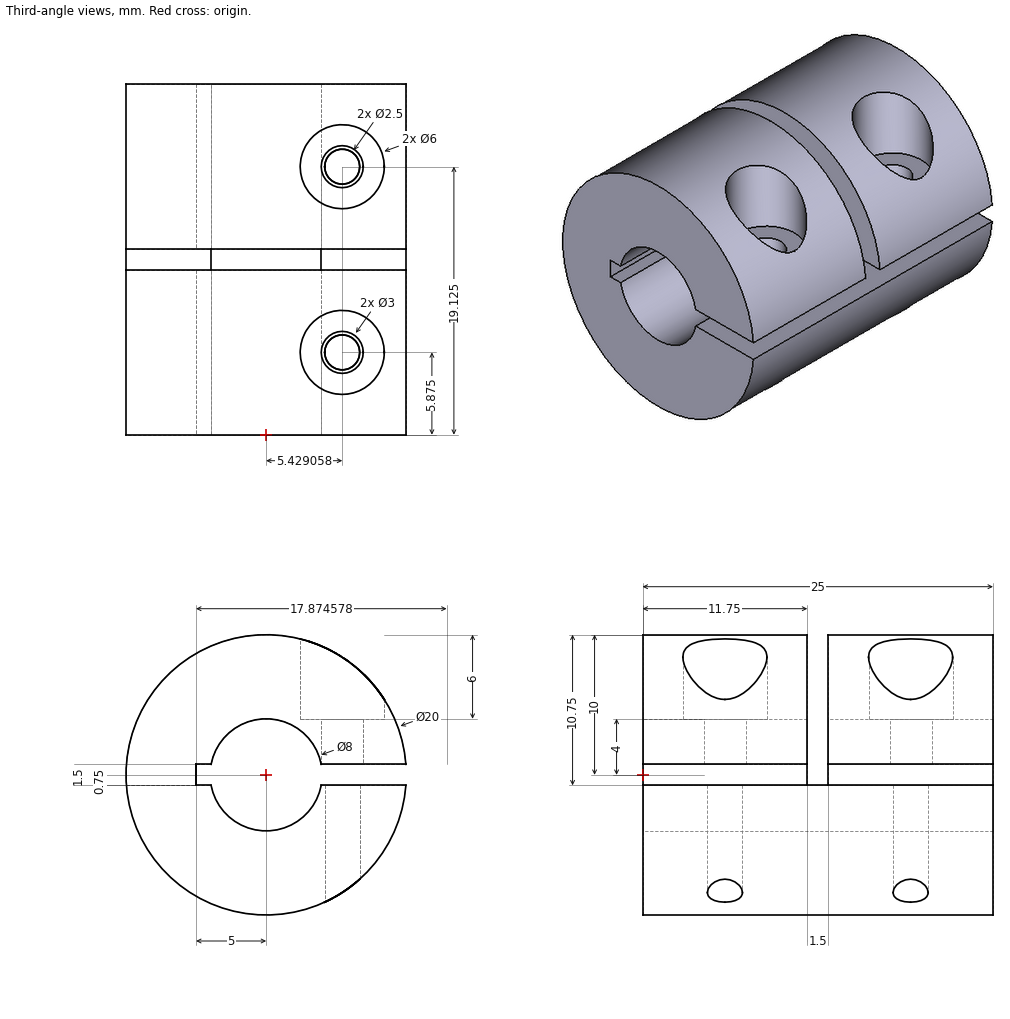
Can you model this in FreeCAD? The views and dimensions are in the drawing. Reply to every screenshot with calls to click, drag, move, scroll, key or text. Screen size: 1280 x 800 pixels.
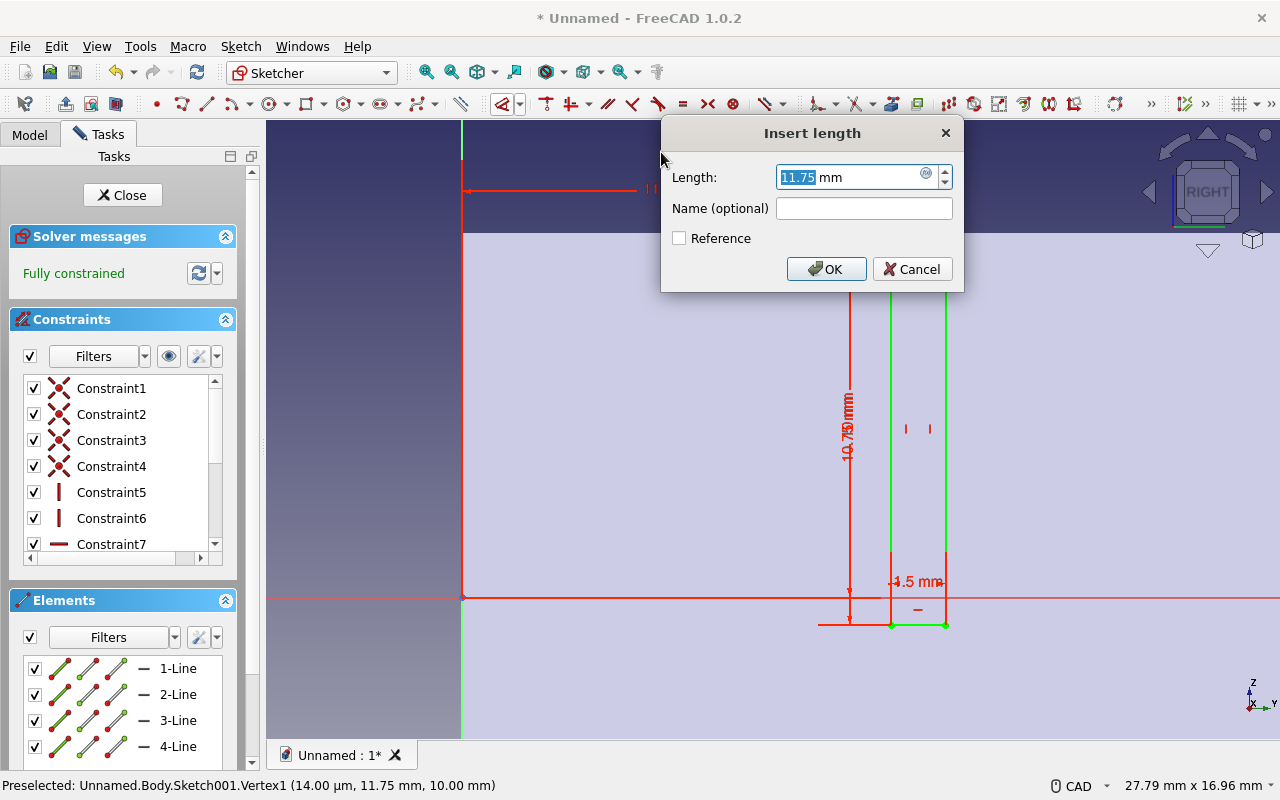
text(11.75)
key(Return)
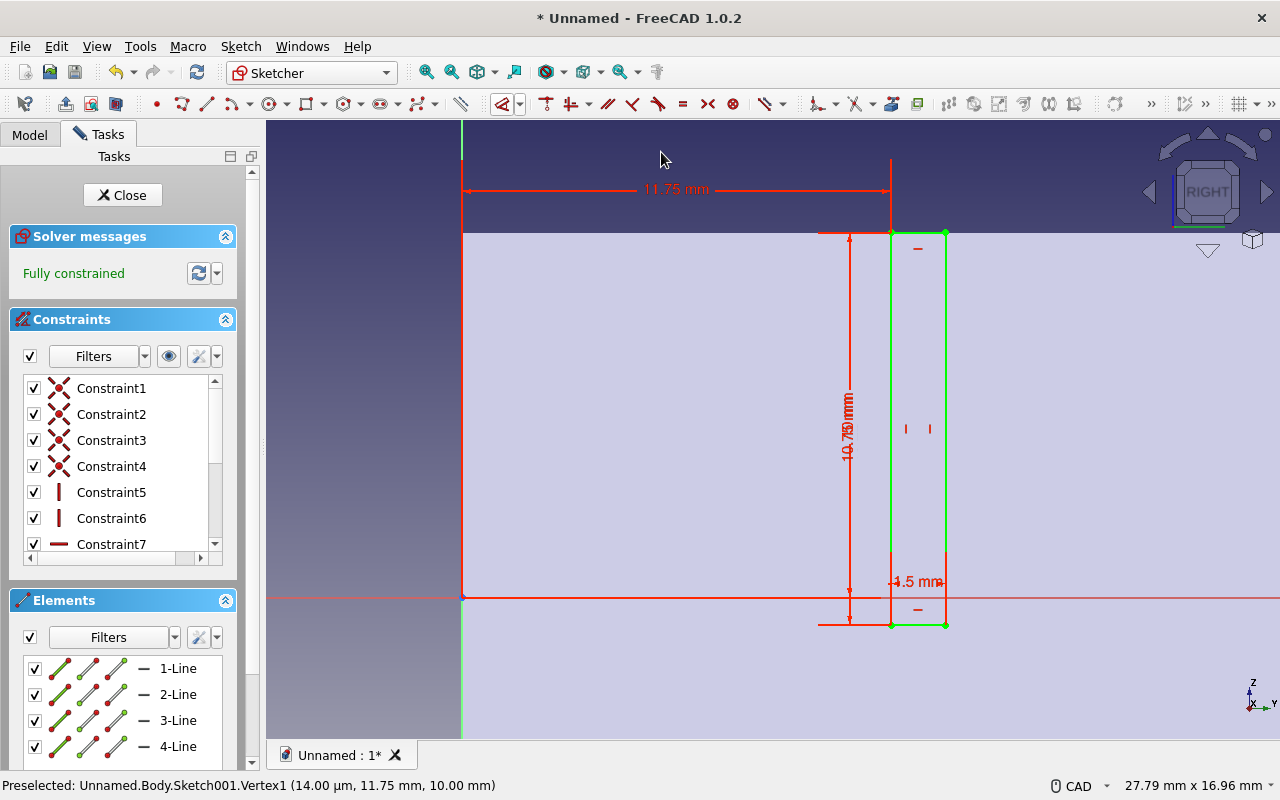
click(123, 195)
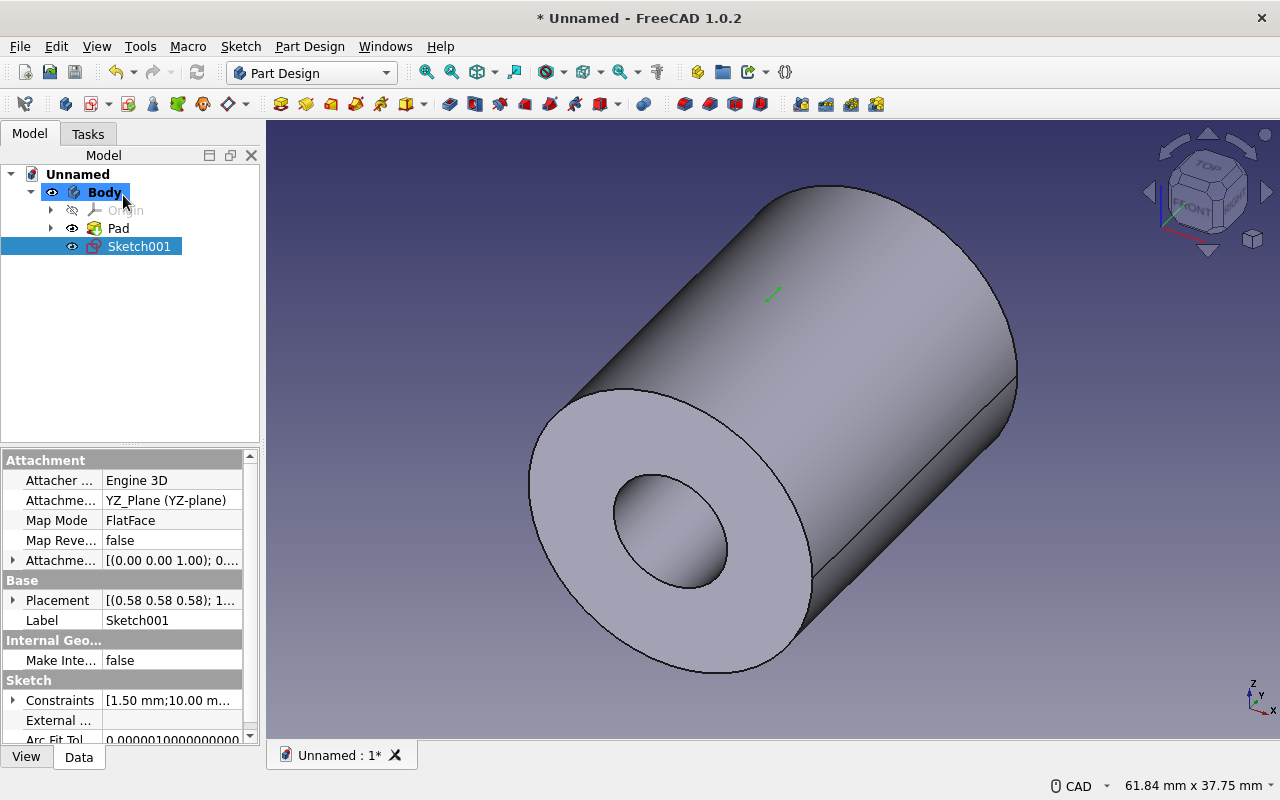
click(450, 104)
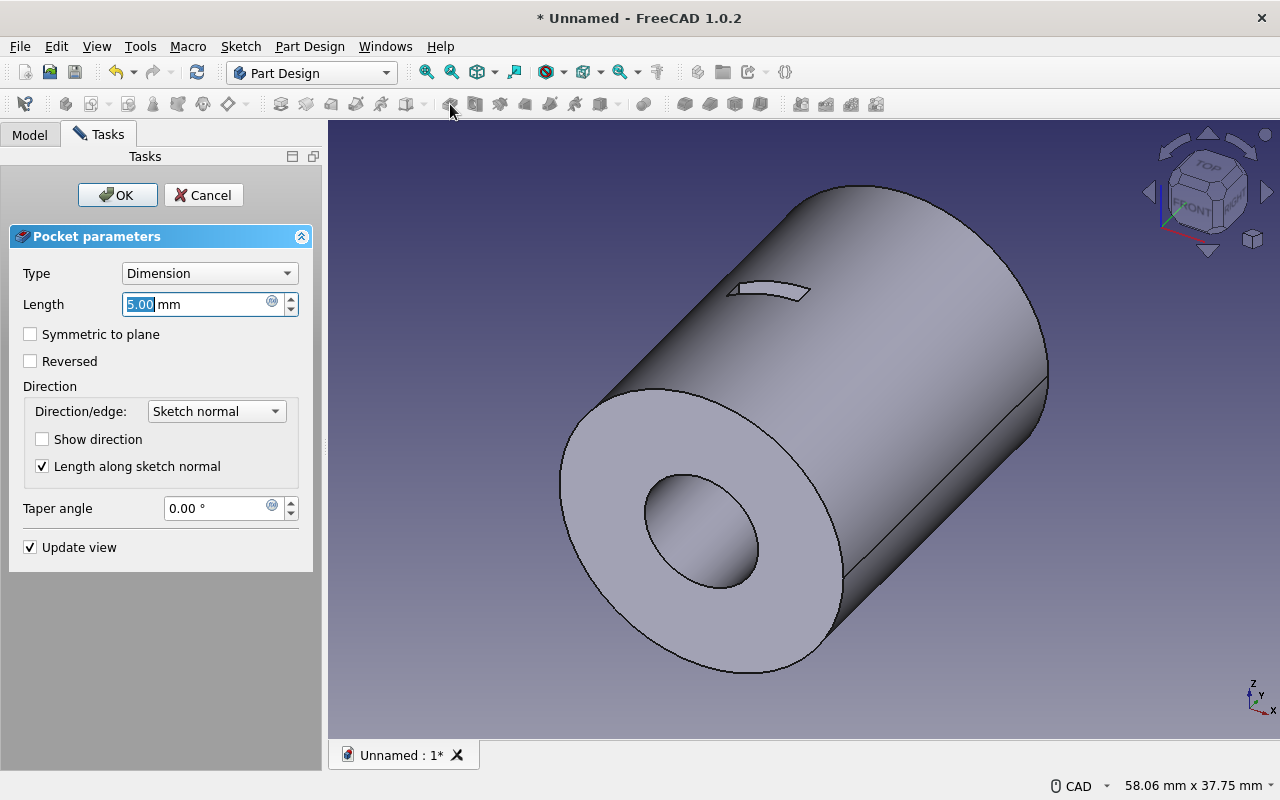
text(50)
key(Tab)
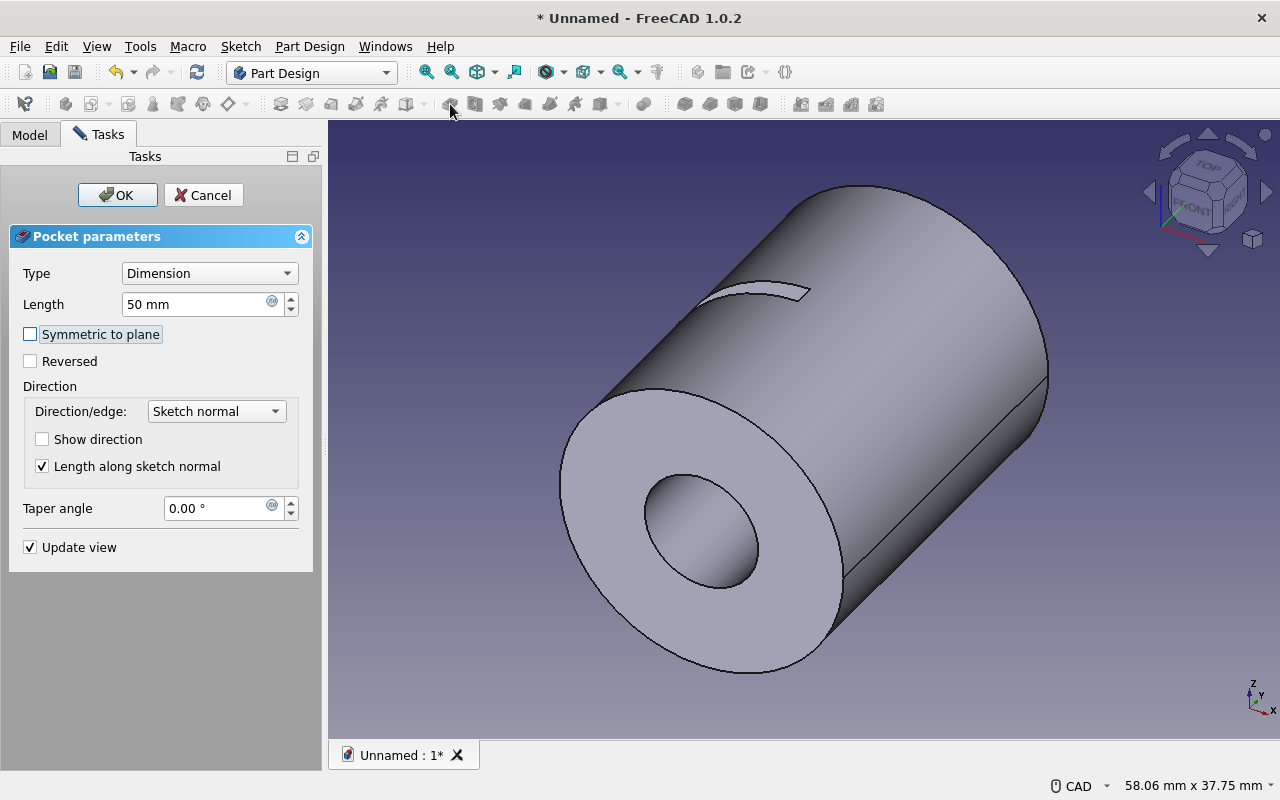
click(31, 334)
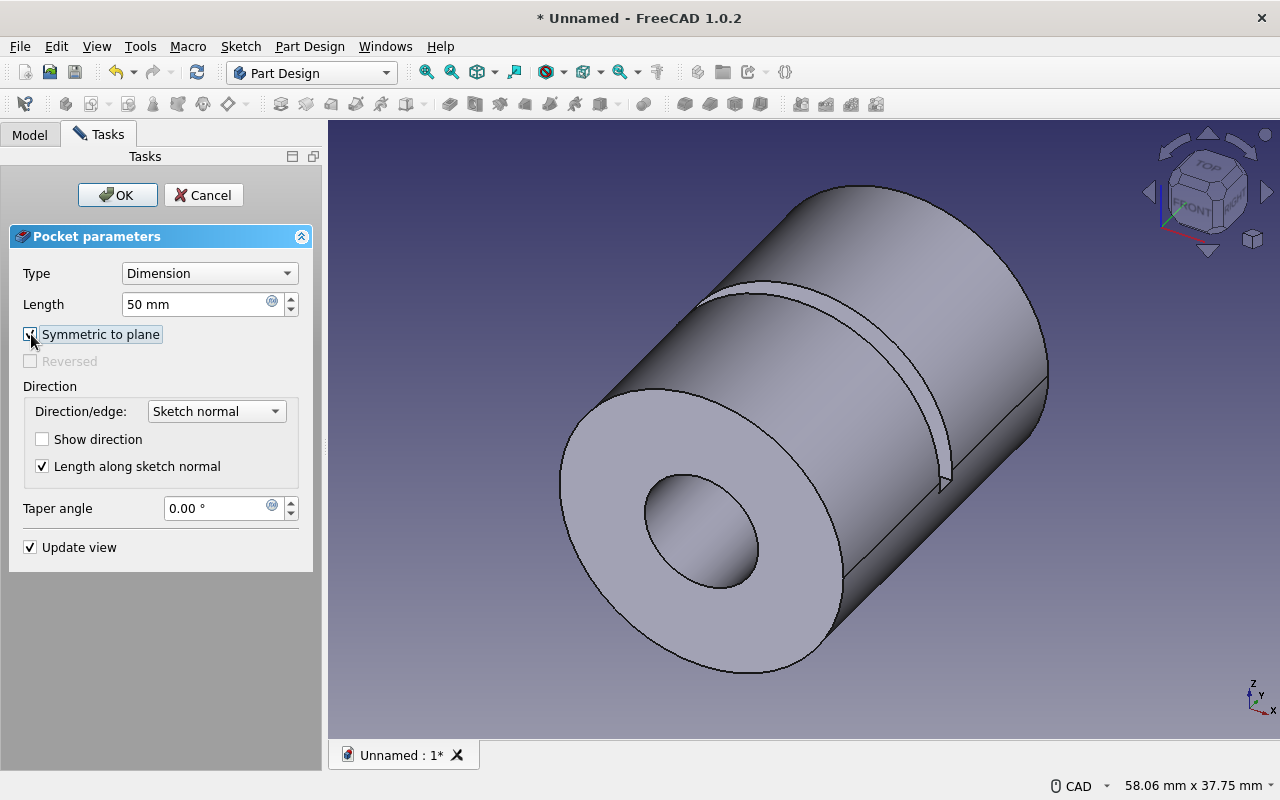
click(118, 195)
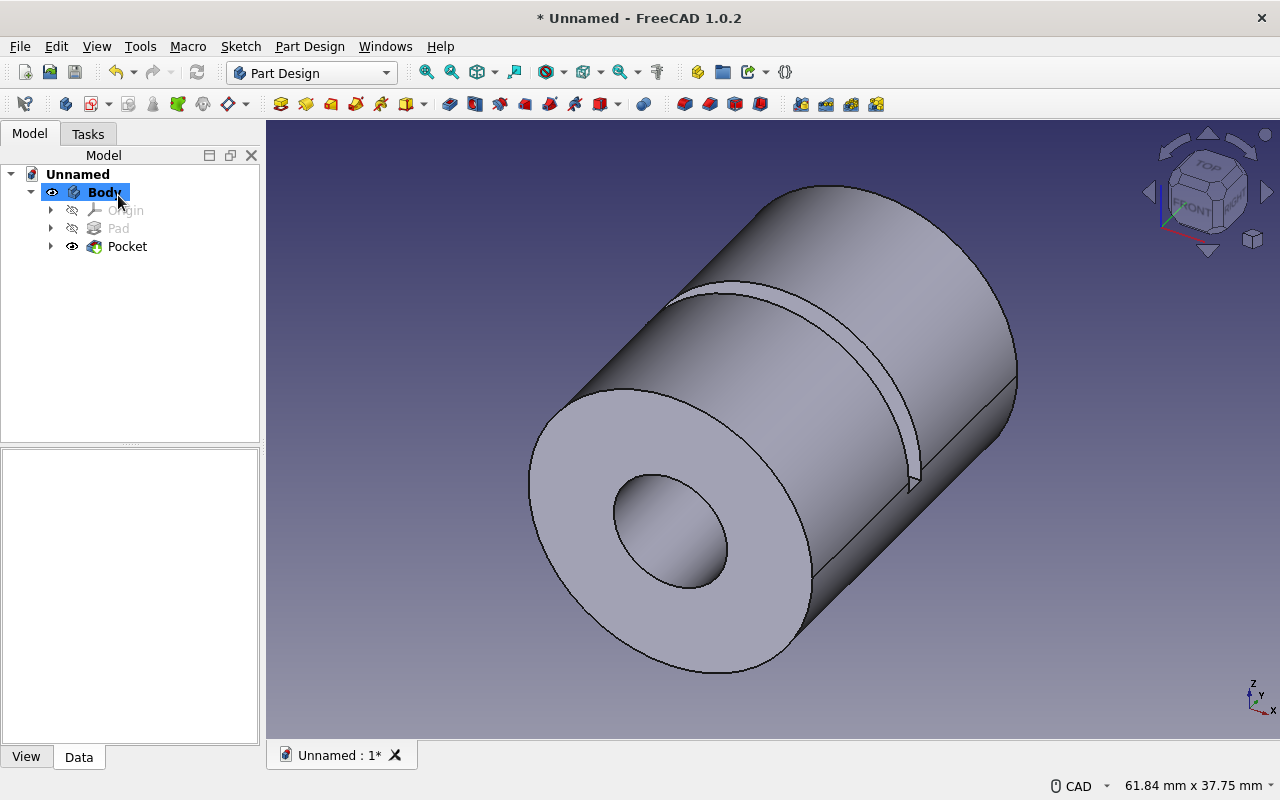
key(4)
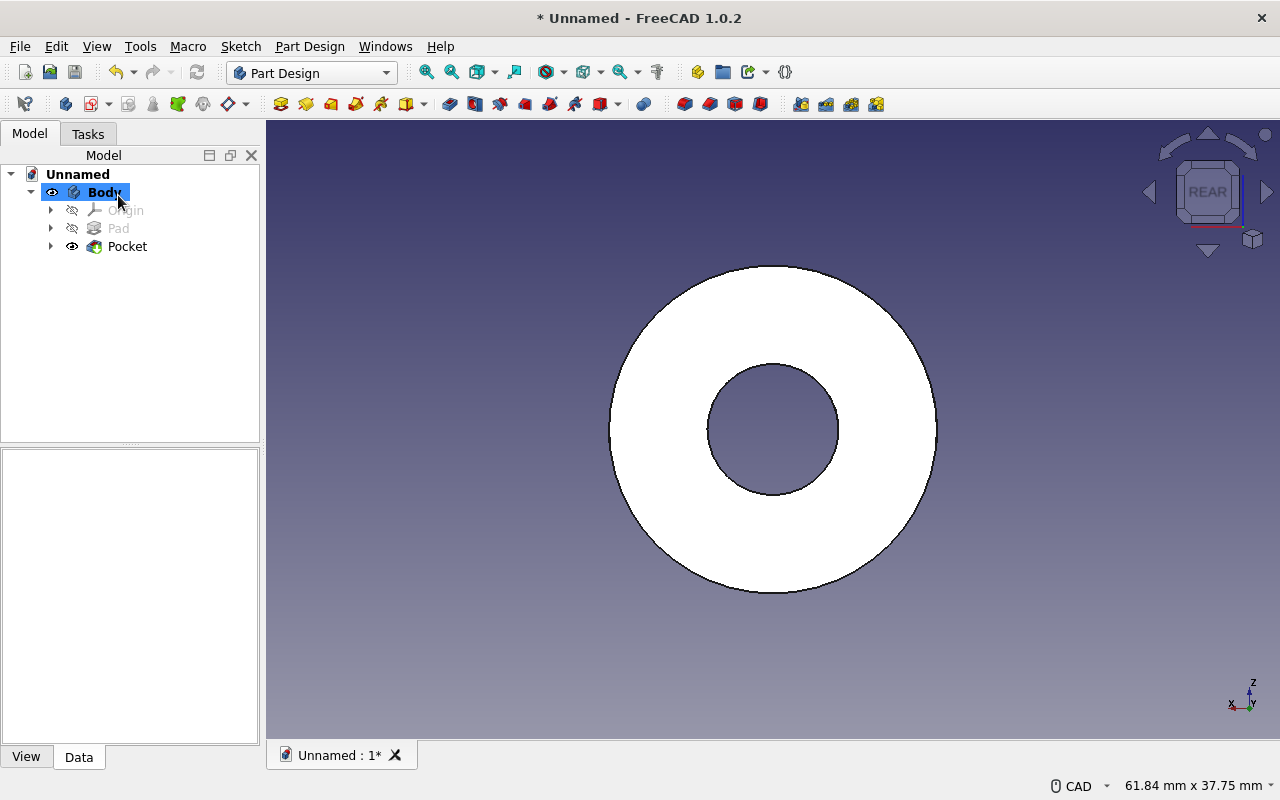
click(867, 382)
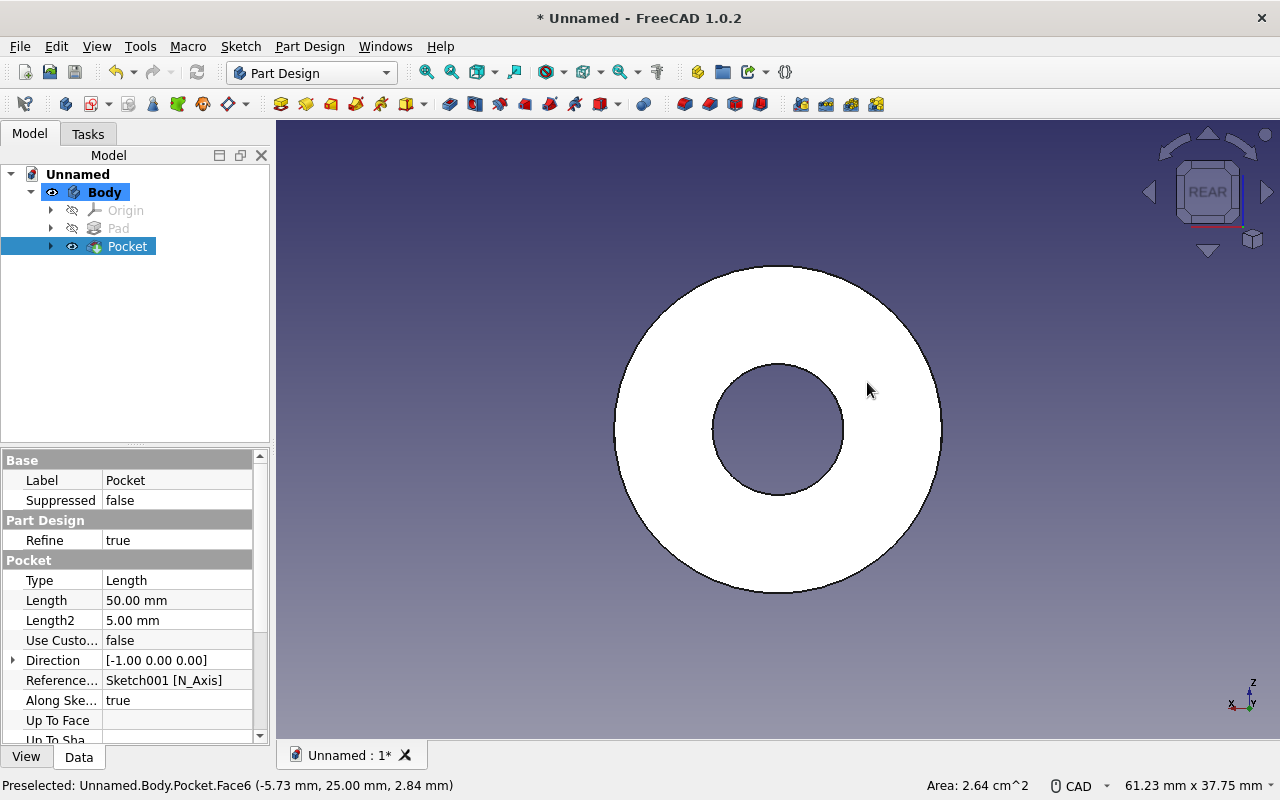
click(90, 104)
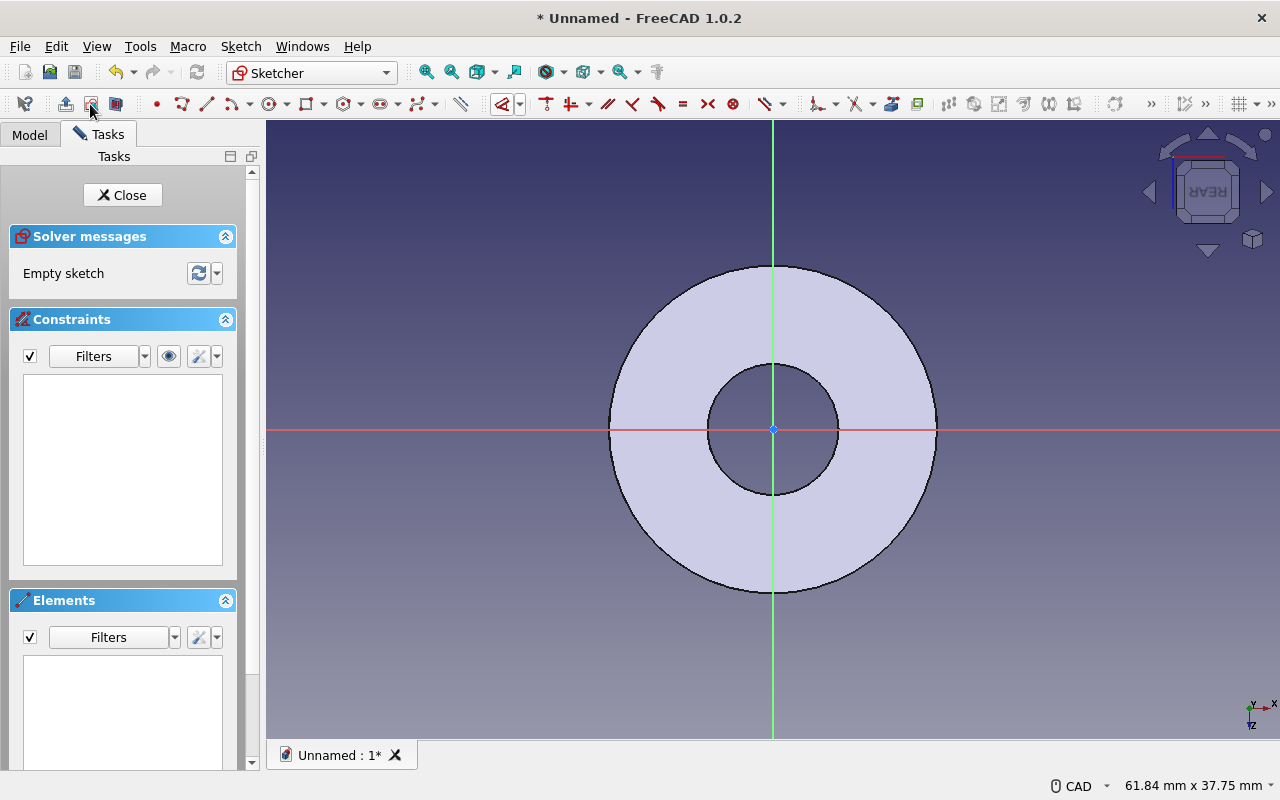
scroll(999, 429, up, 3)